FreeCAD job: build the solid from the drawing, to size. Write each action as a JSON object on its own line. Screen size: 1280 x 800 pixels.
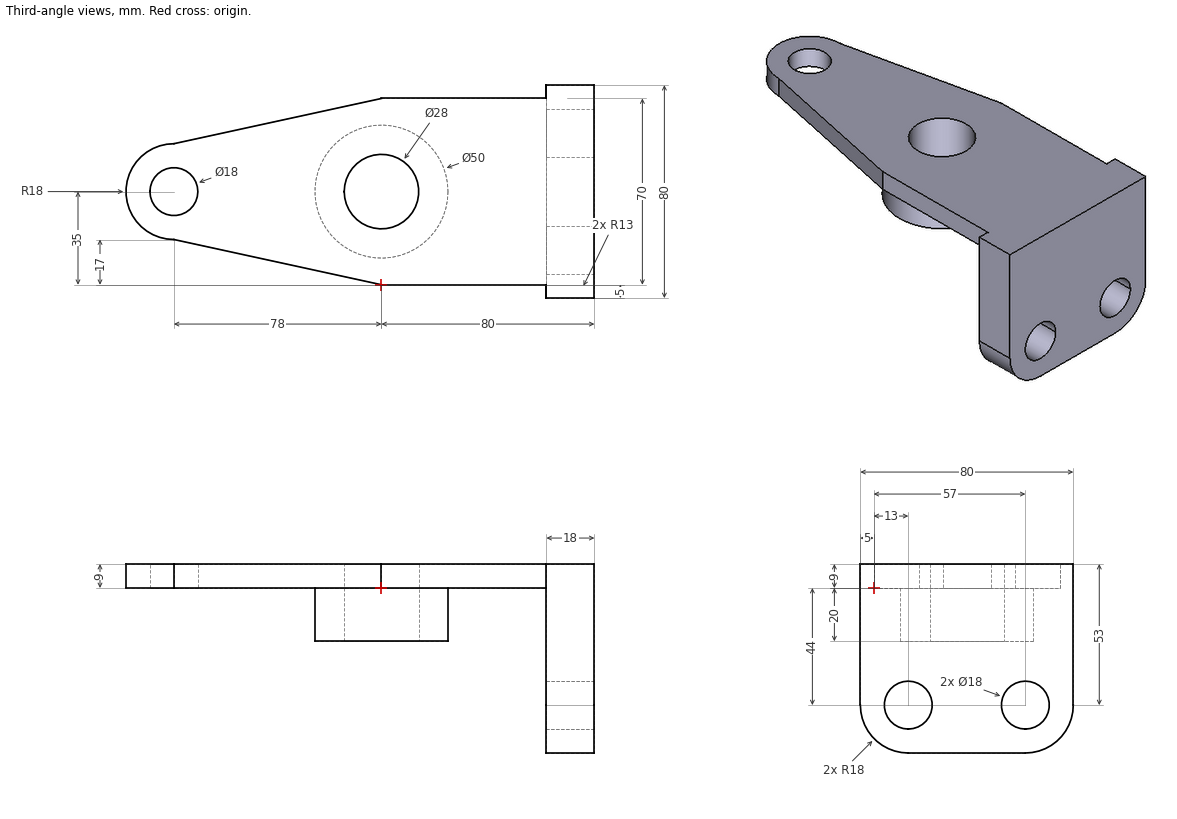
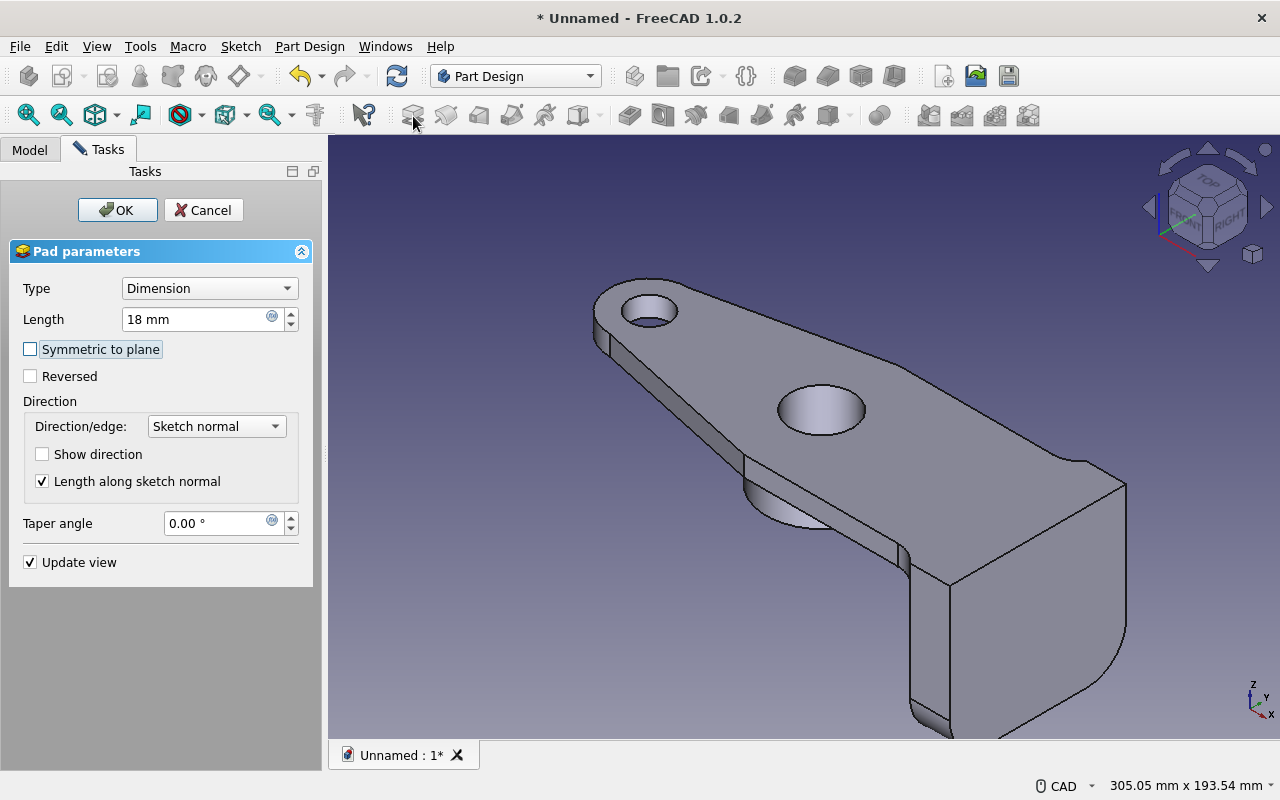
{"action": "left_click", "coordinate": [31, 376]}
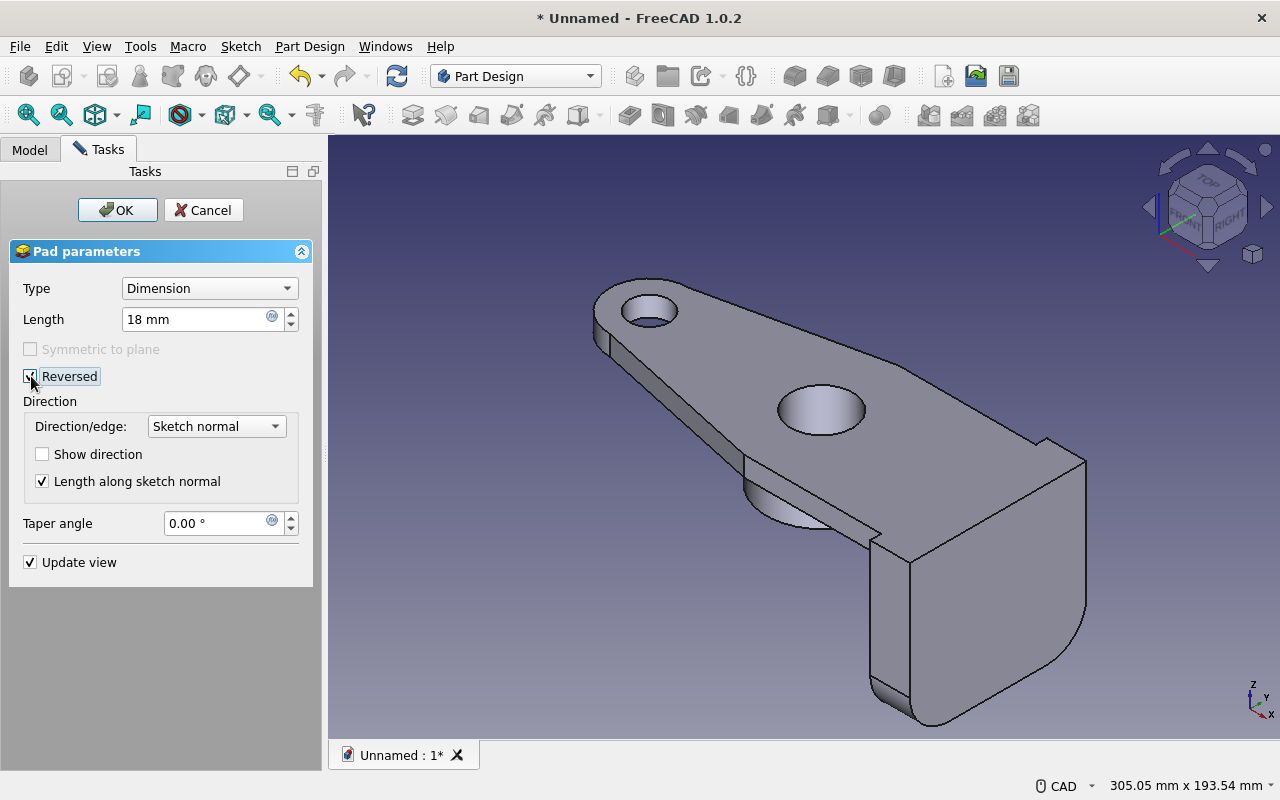
{"action": "left_click", "coordinate": [118, 210]}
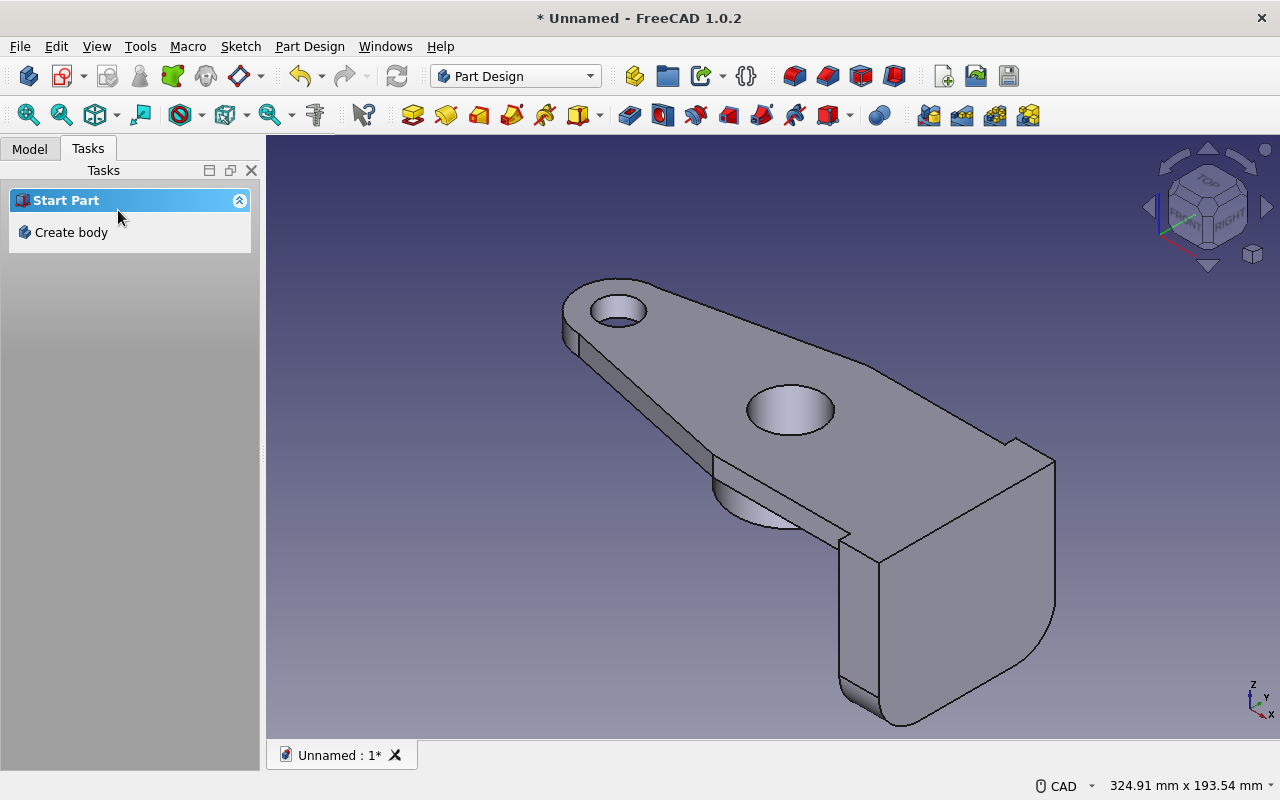
{"action": "left_click", "coordinate": [29, 116]}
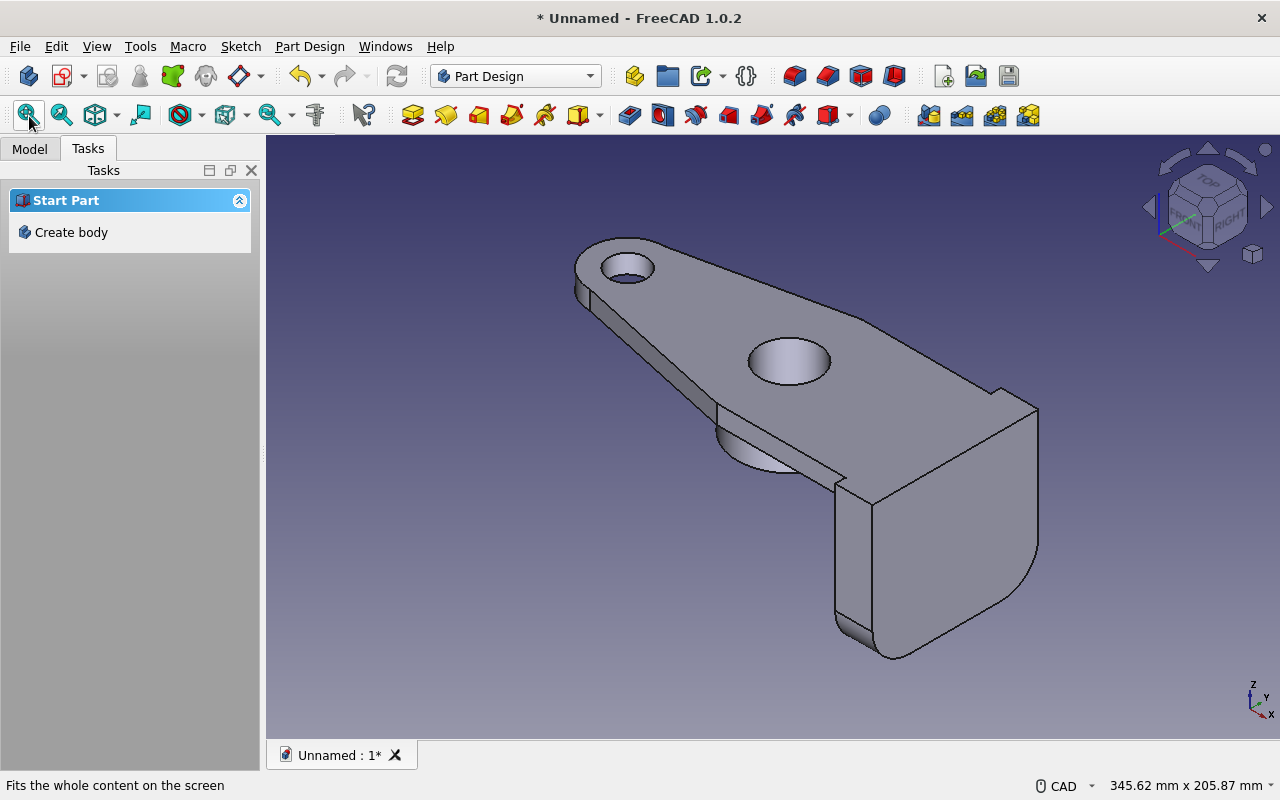
{"action": "left_click", "coordinate": [955, 541]}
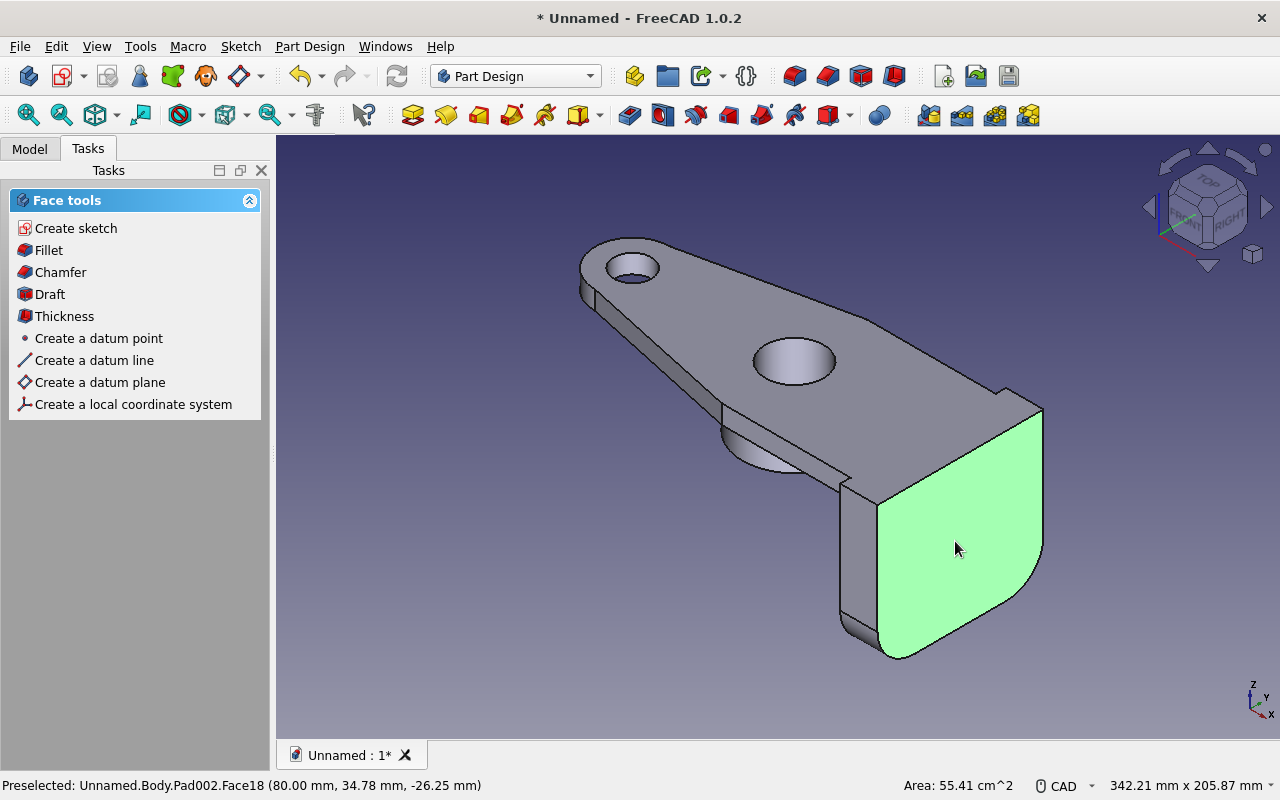
{"action": "left_click", "coordinate": [62, 76]}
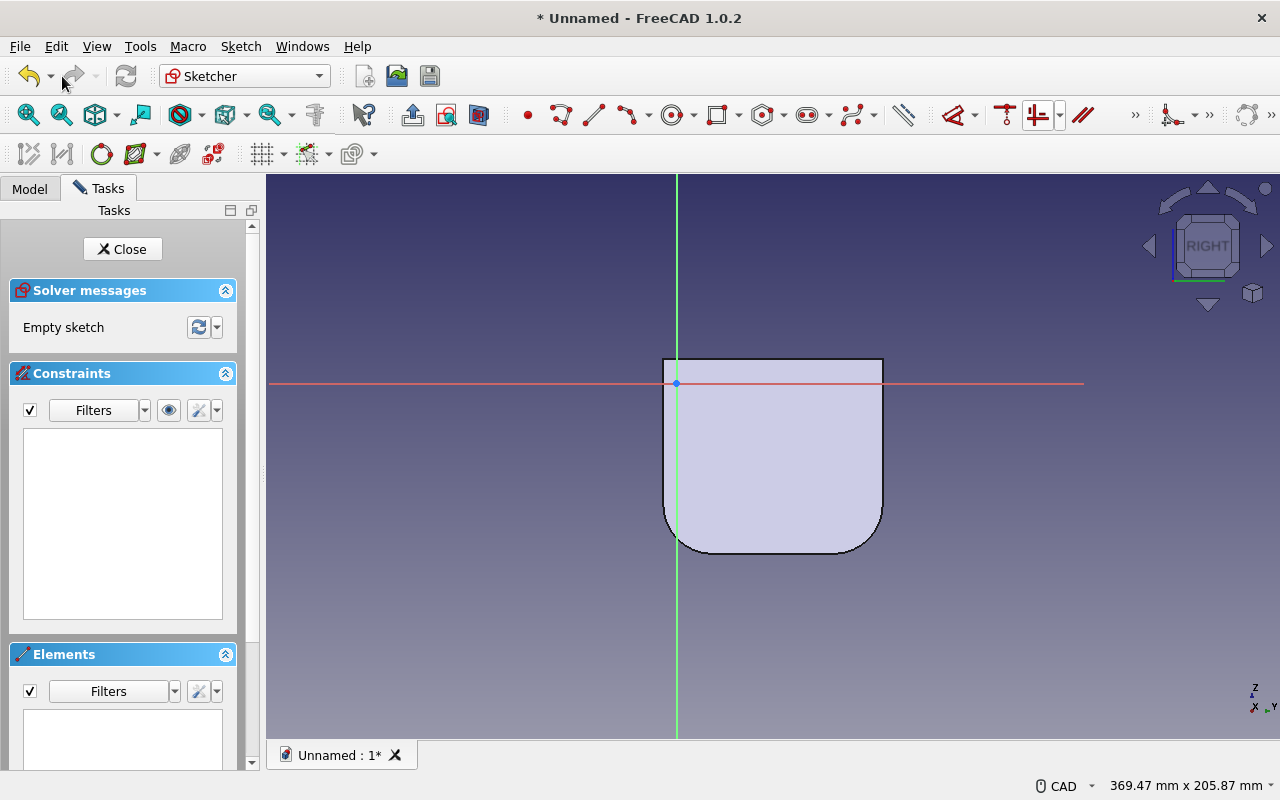
{"action": "scroll", "coordinate": [804, 456], "scroll_direction": "up", "scroll_amount": 5}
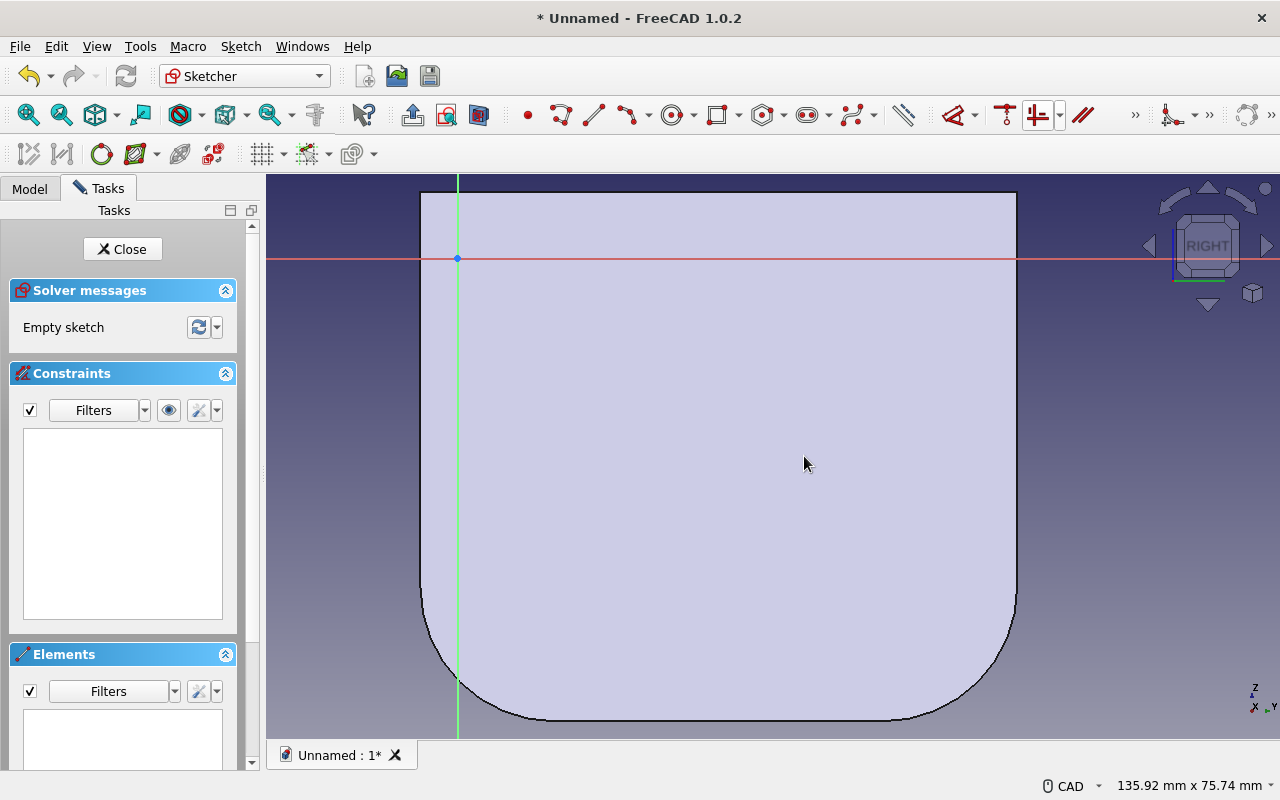
{"action": "left_click", "coordinate": [672, 116]}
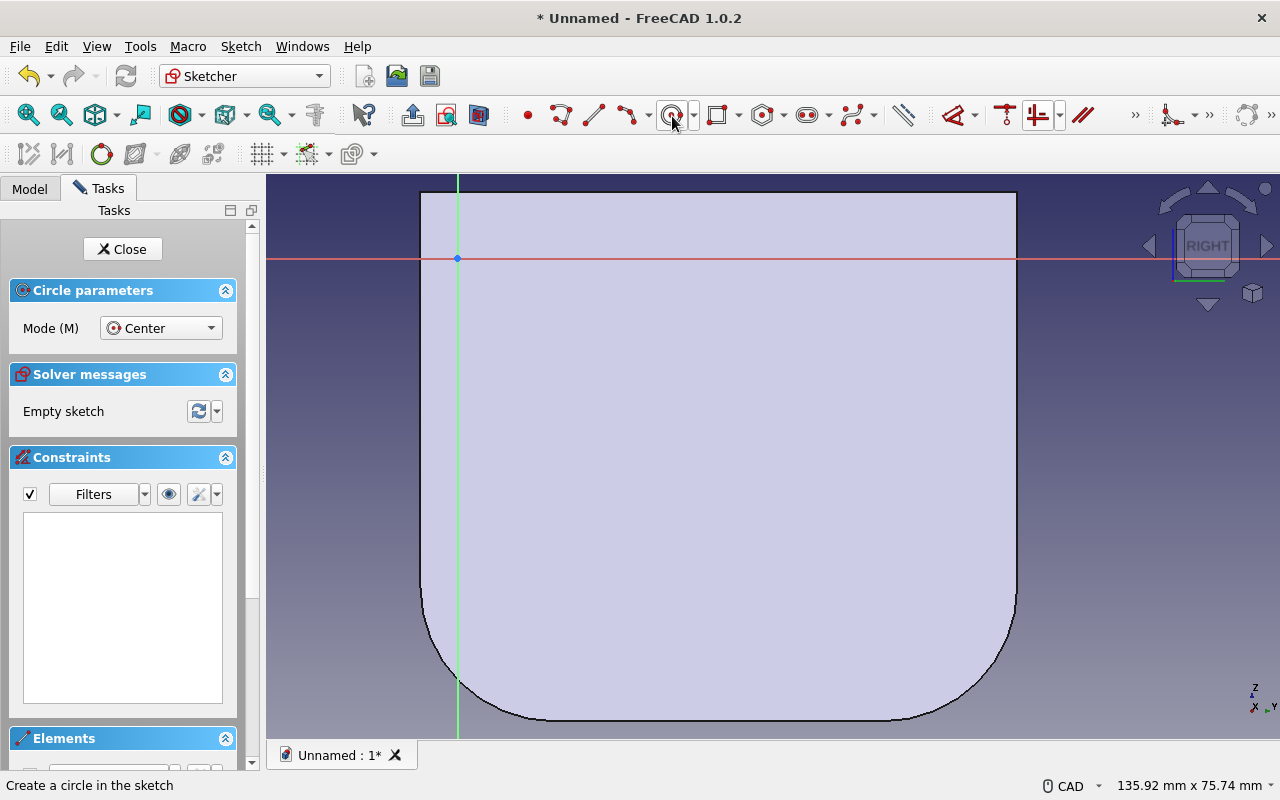
{"action": "left_click", "coordinate": [883, 587]}
{"action": "left_click", "coordinate": [930, 540]}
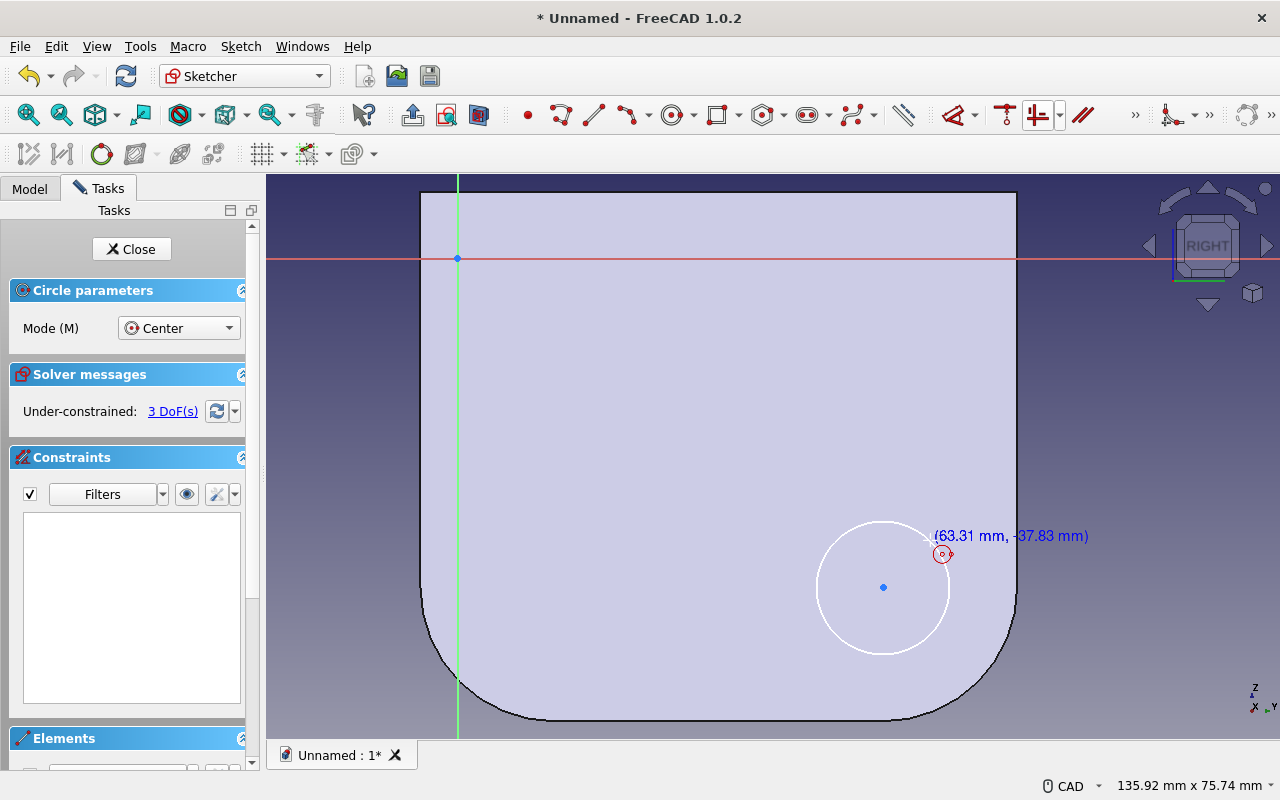
{"action": "left_click", "coordinate": [555, 587]}
{"action": "left_click", "coordinate": [602, 540]}
{"action": "key", "text": "Escape"}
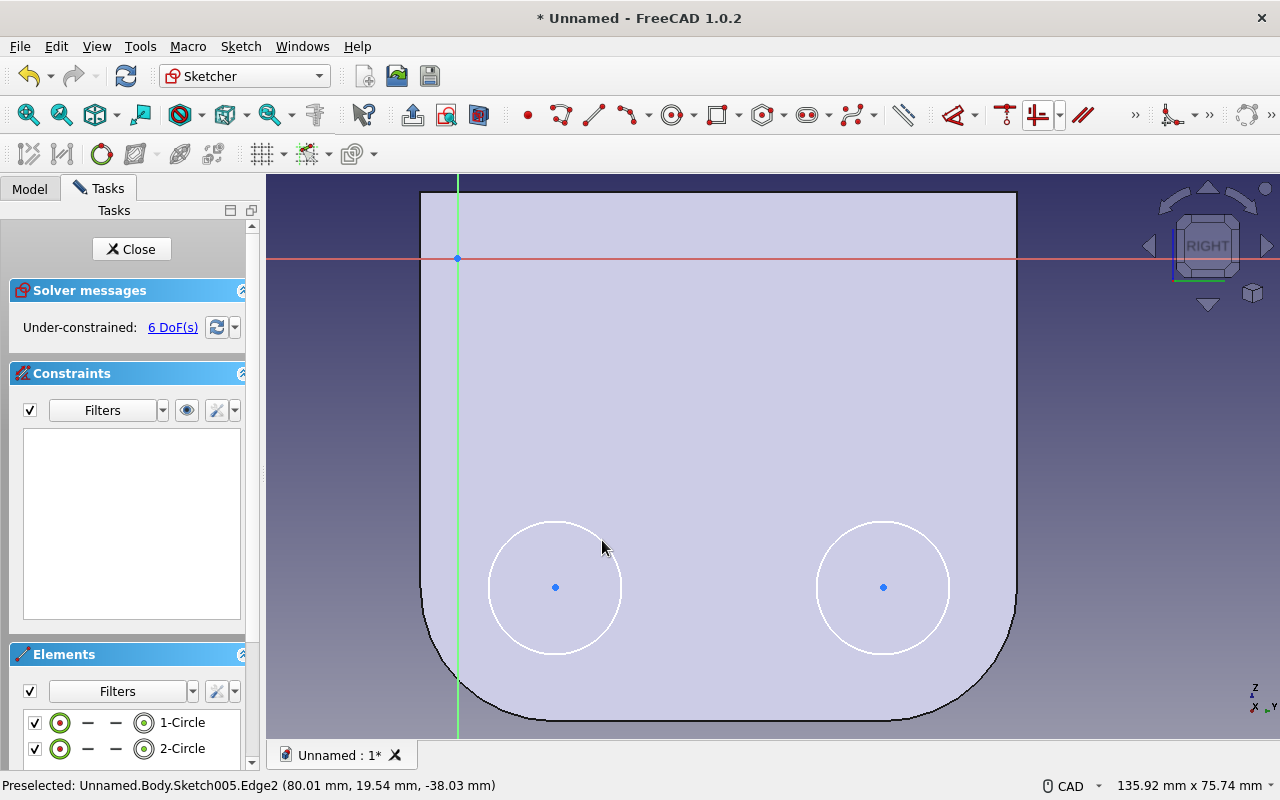
{"action": "left_click", "coordinate": [930, 541]}